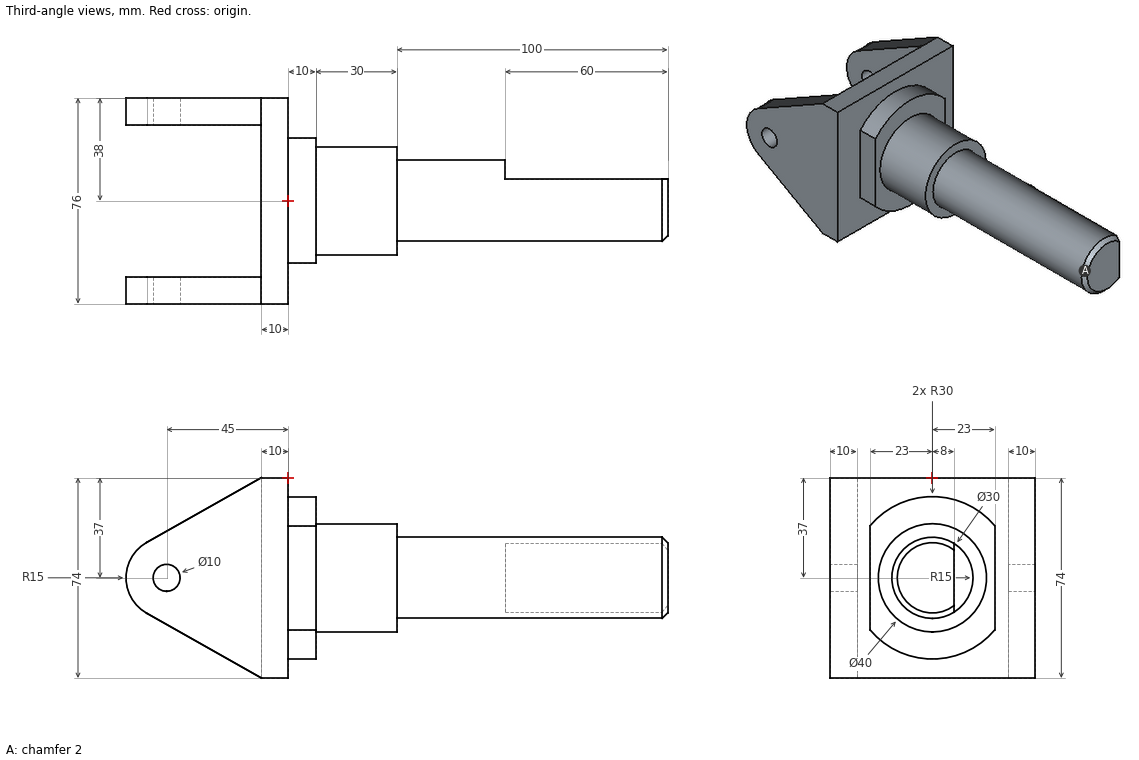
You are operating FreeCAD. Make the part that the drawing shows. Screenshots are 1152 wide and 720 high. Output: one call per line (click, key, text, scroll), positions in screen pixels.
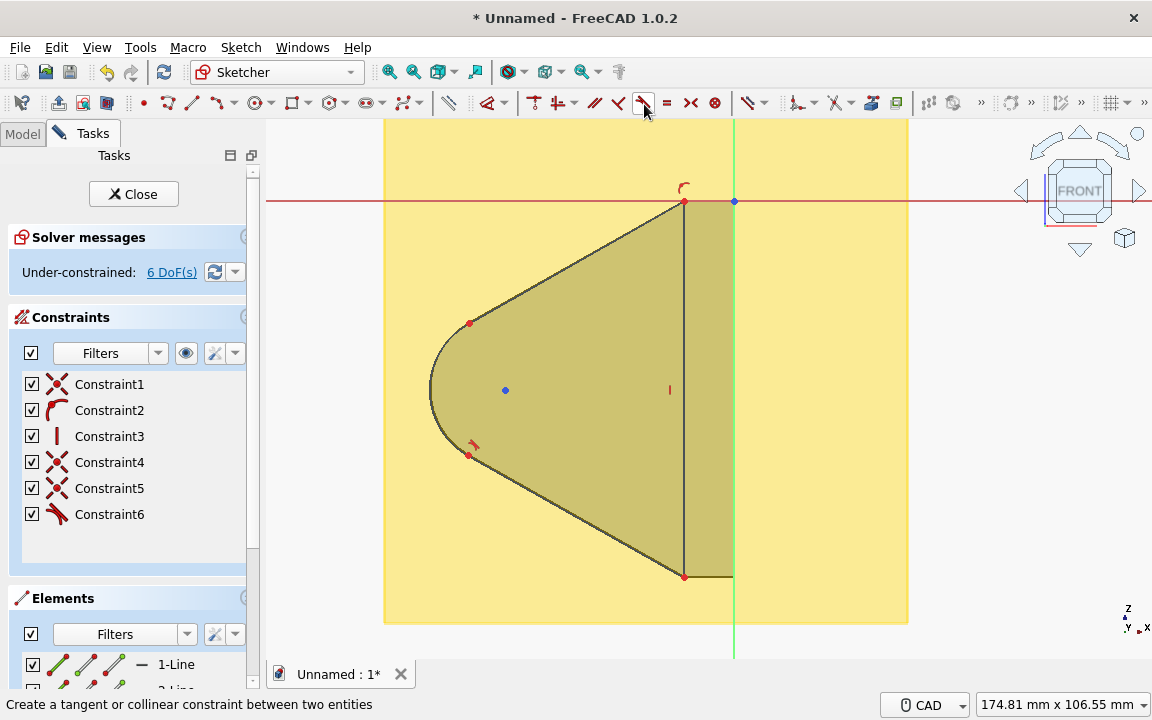
click(620, 238)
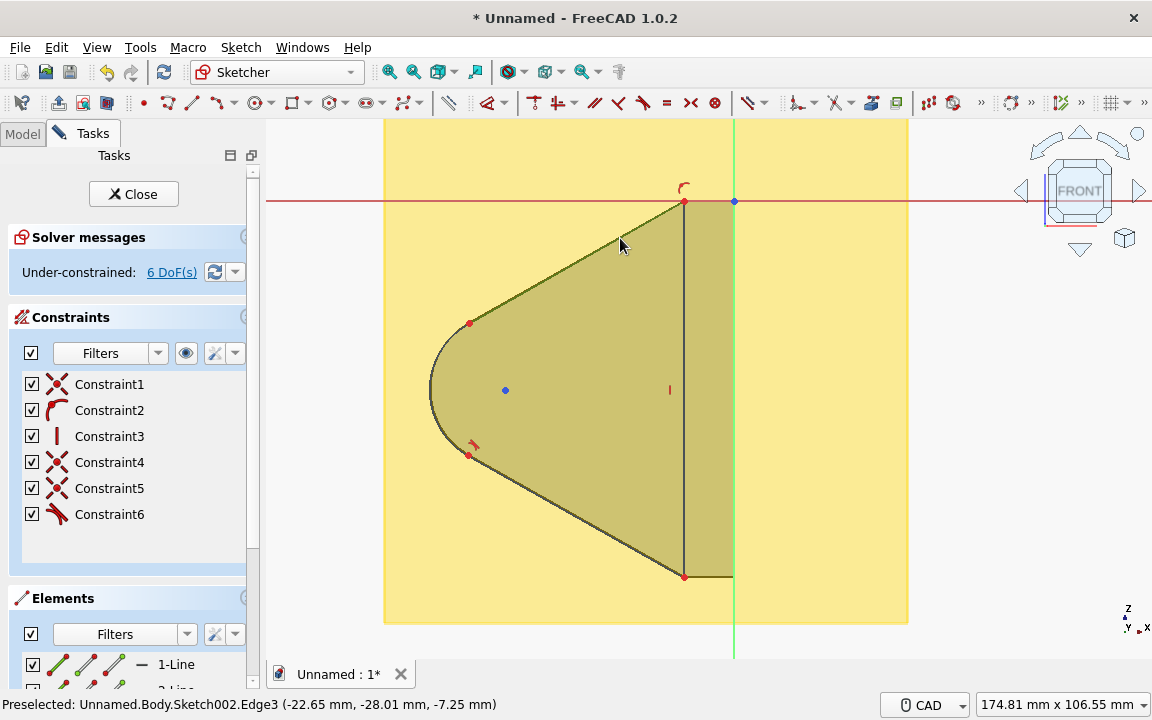
click(437, 359)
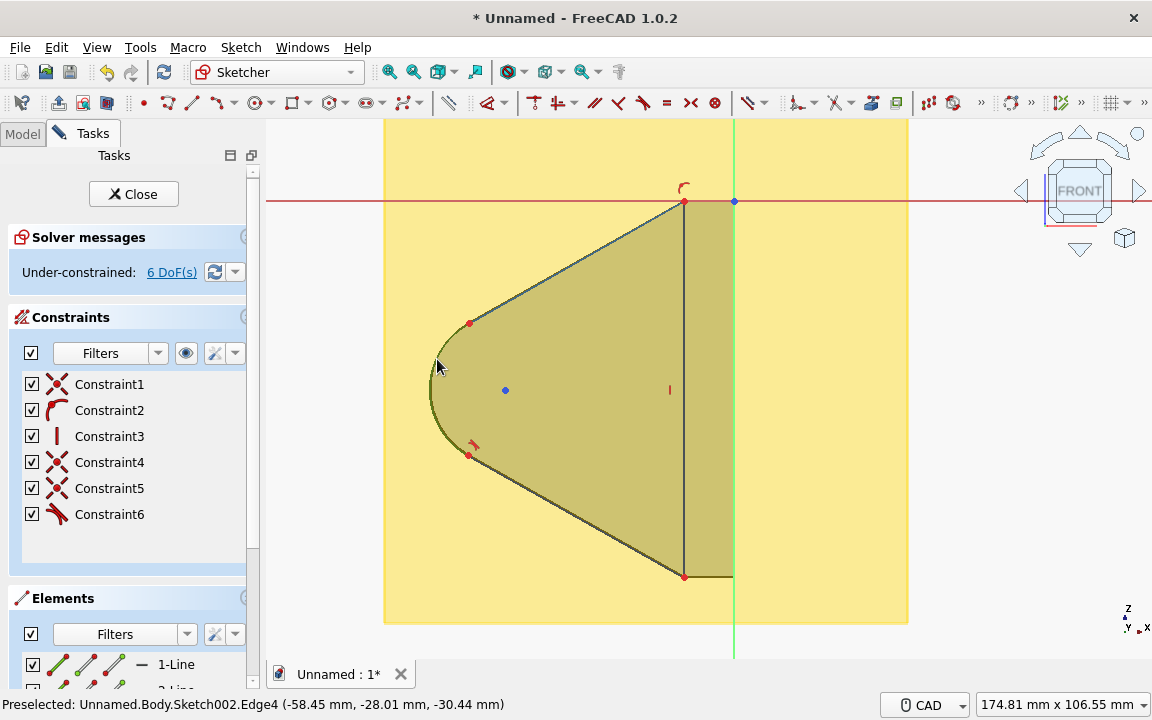
click(644, 104)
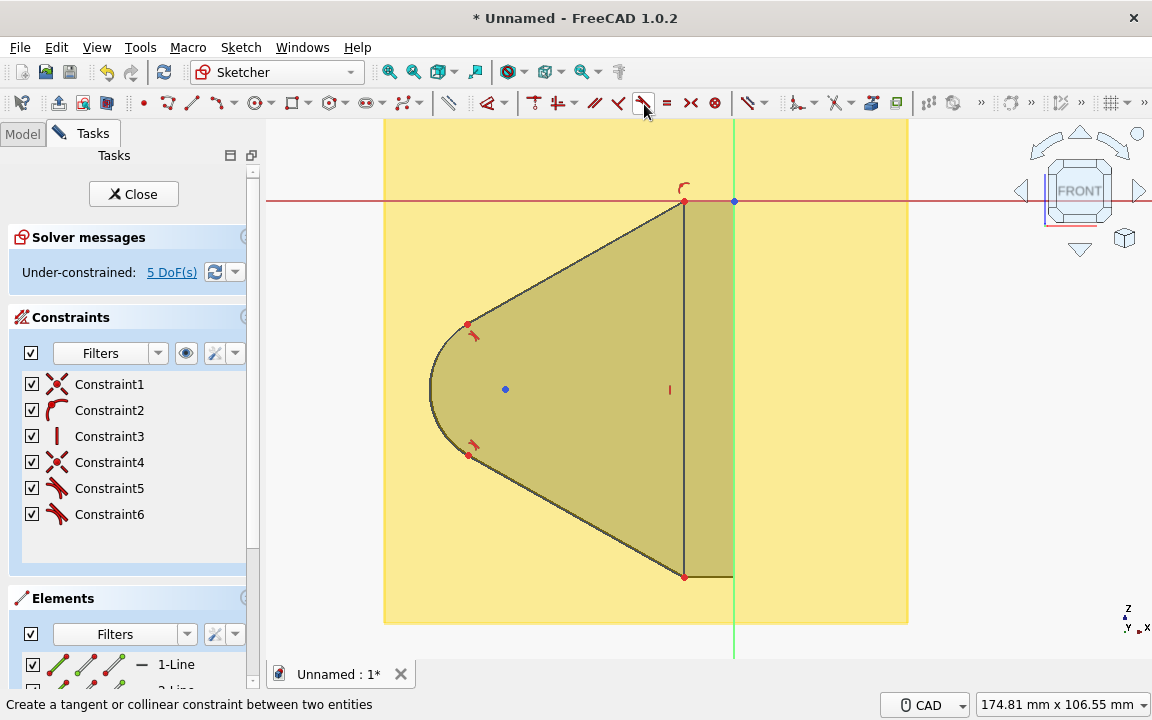
click(488, 104)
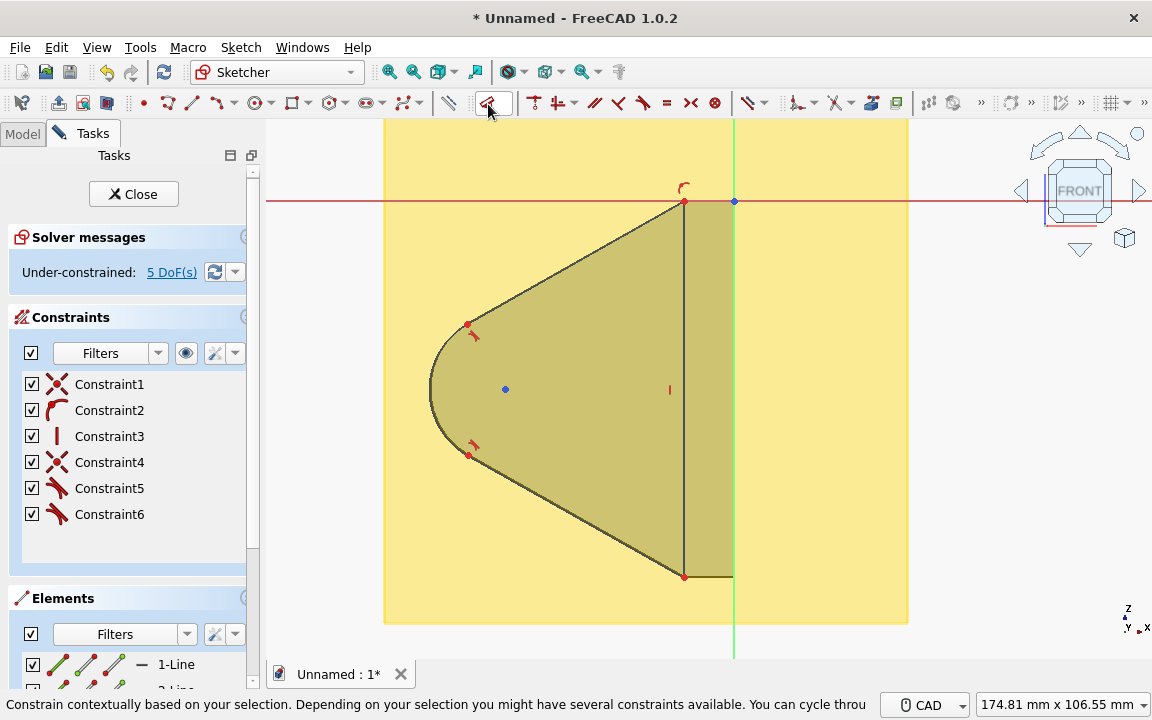
click(436, 359)
click(407, 346)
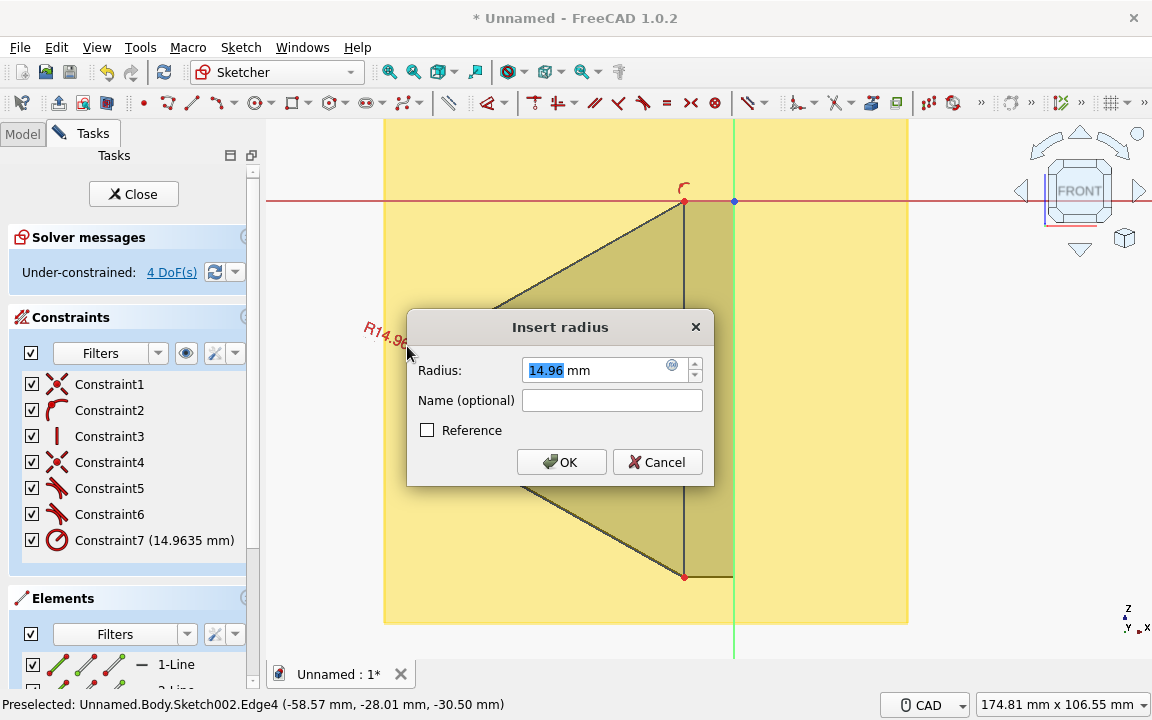
text(15)
key(Return)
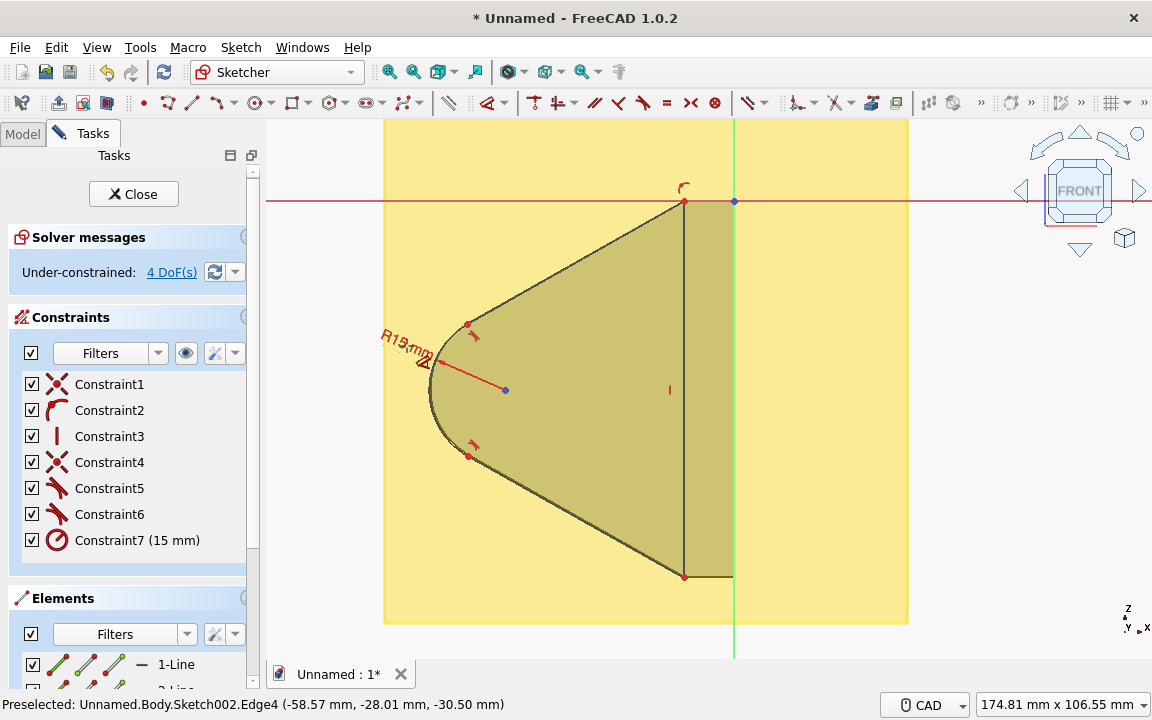
click(684, 465)
click(718, 390)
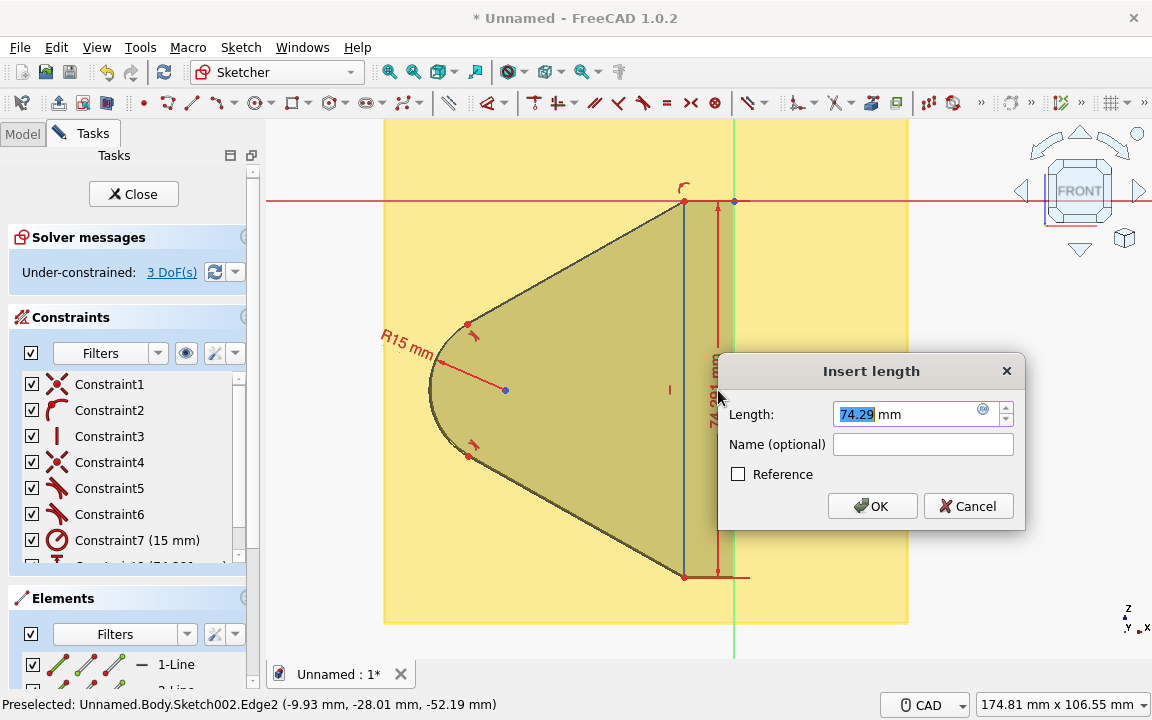
text(74)
key(Return)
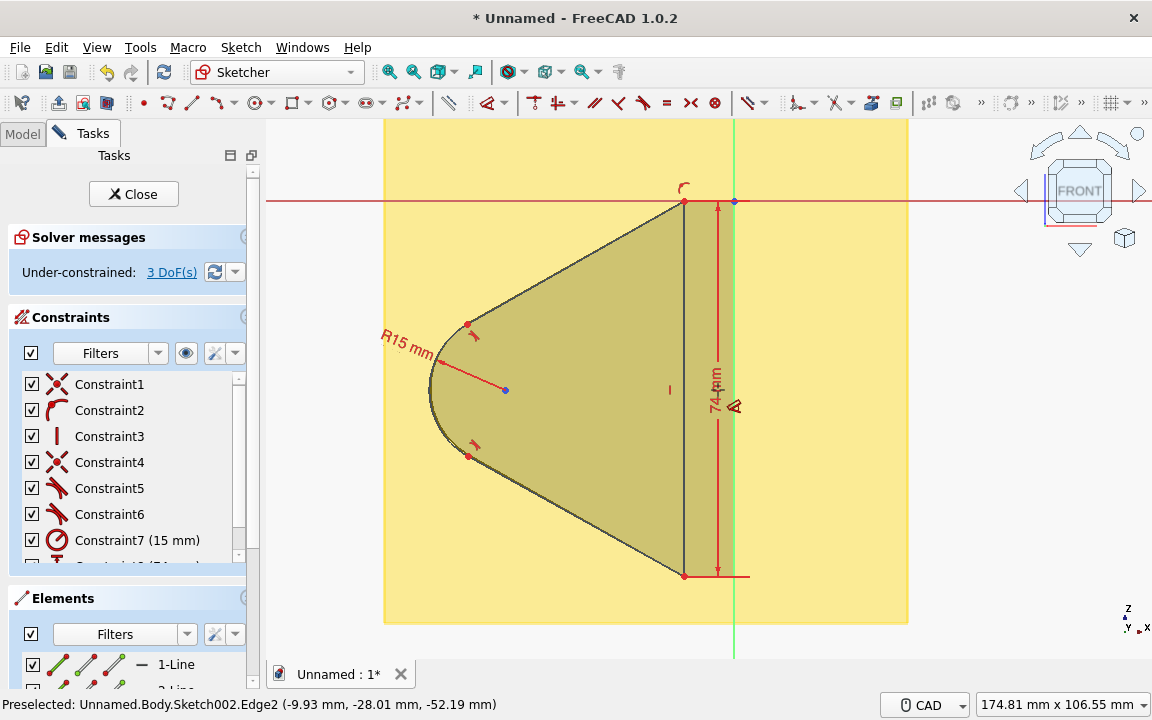
click(684, 577)
click(709, 611)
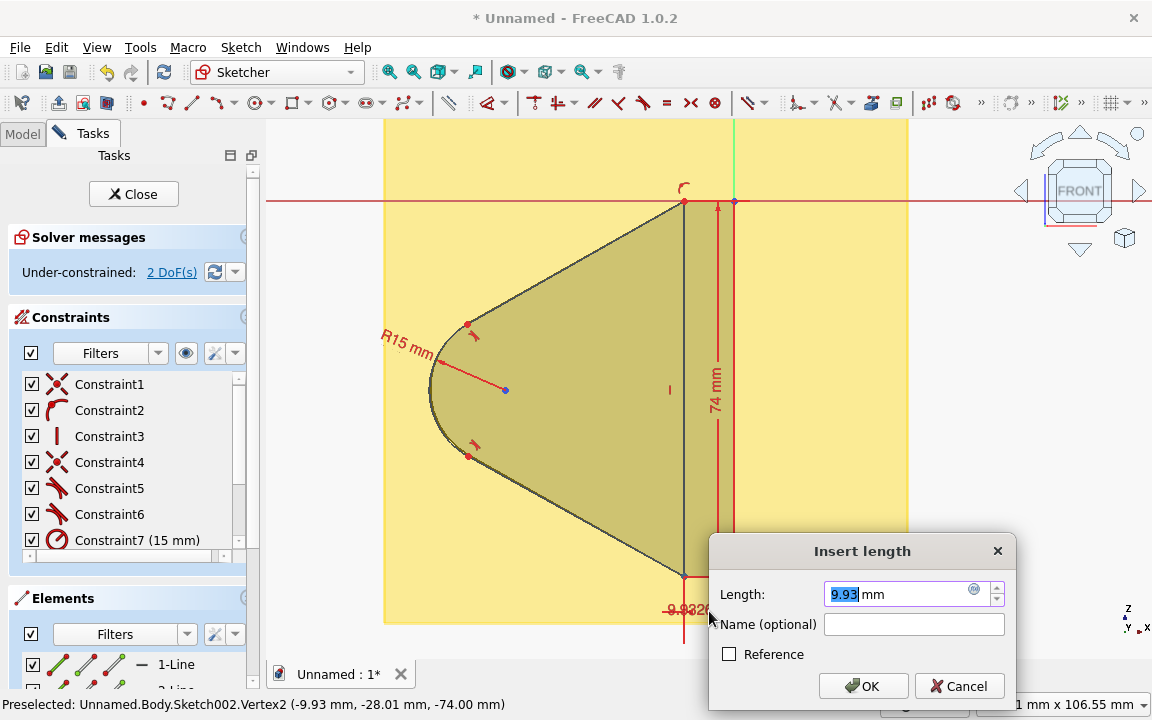
text(10)
key(Return)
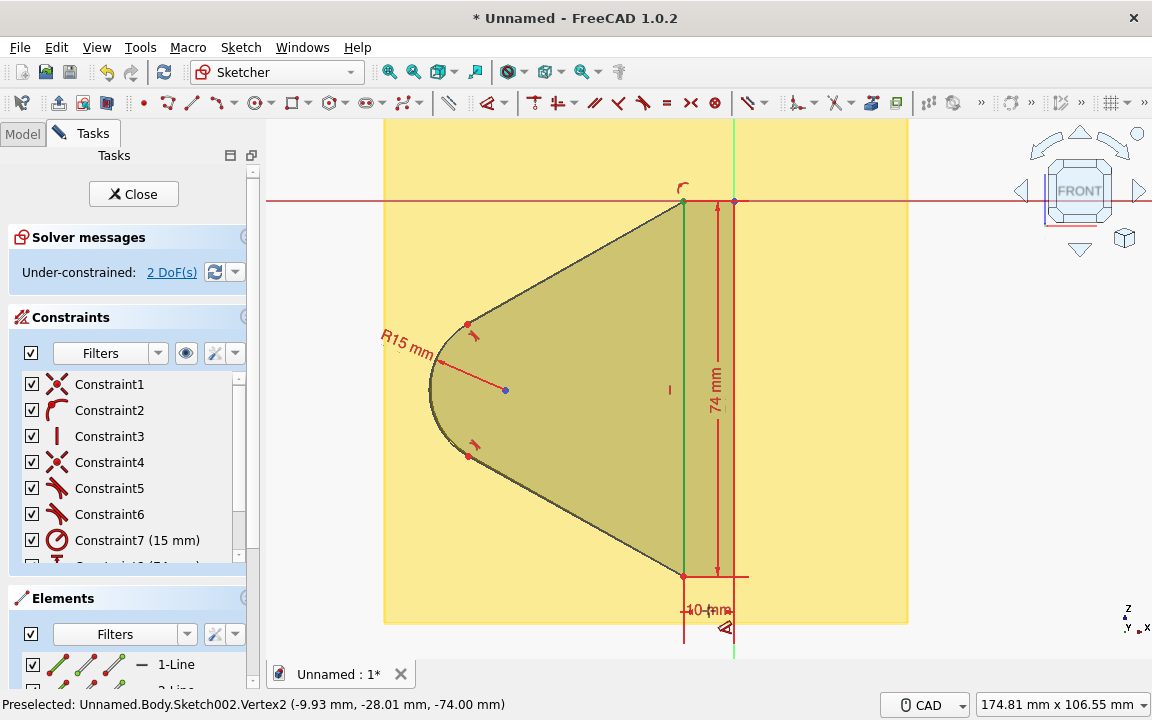
click(505, 390)
click(620, 167)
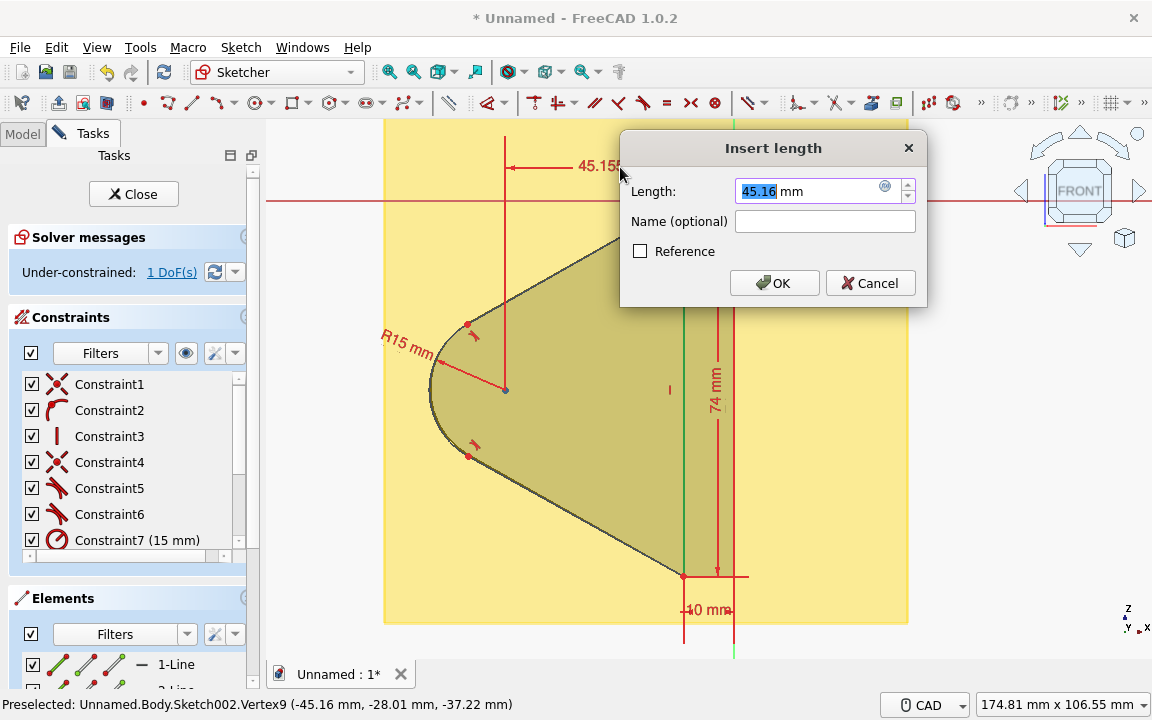
text(45)
key(Return)